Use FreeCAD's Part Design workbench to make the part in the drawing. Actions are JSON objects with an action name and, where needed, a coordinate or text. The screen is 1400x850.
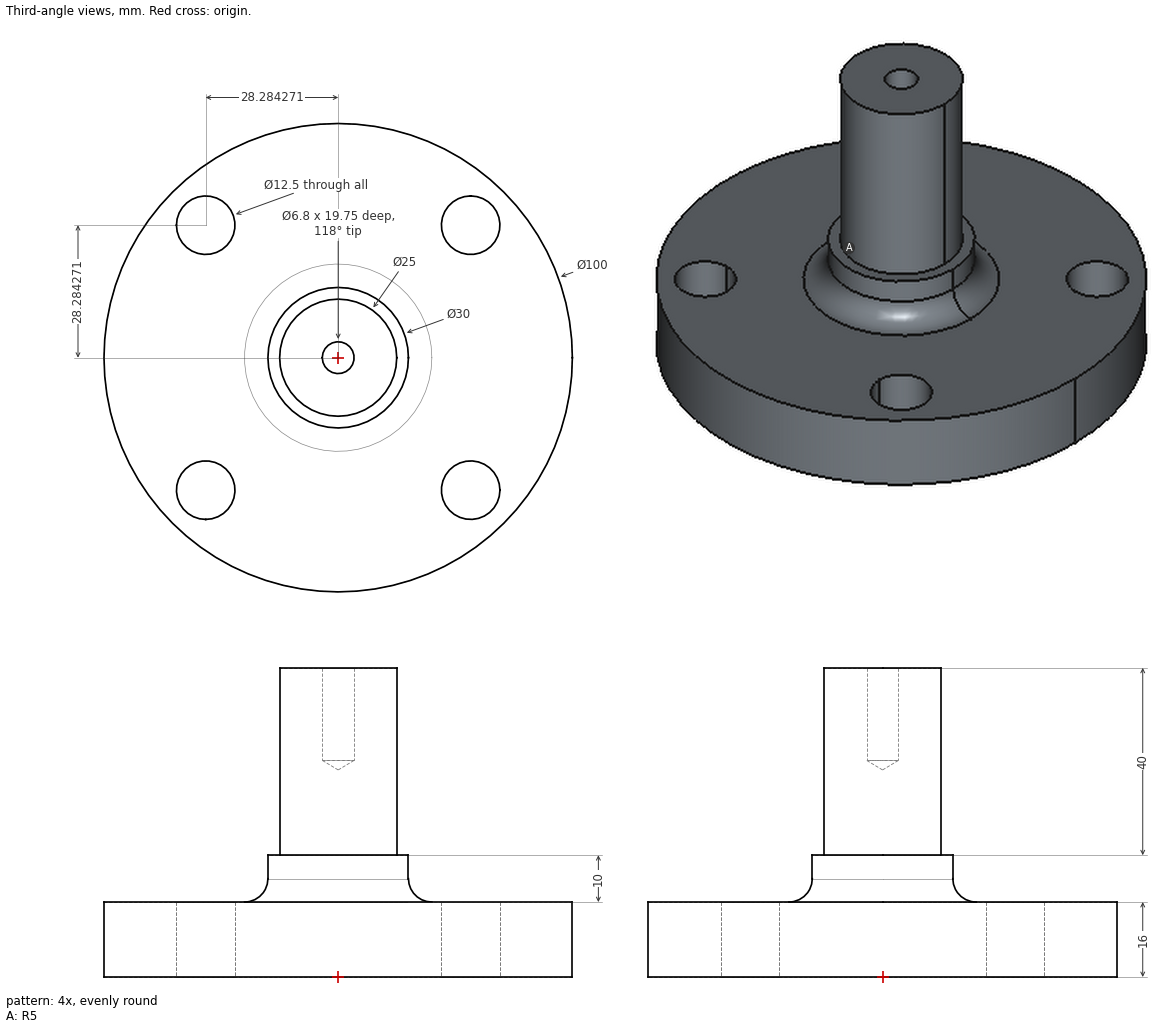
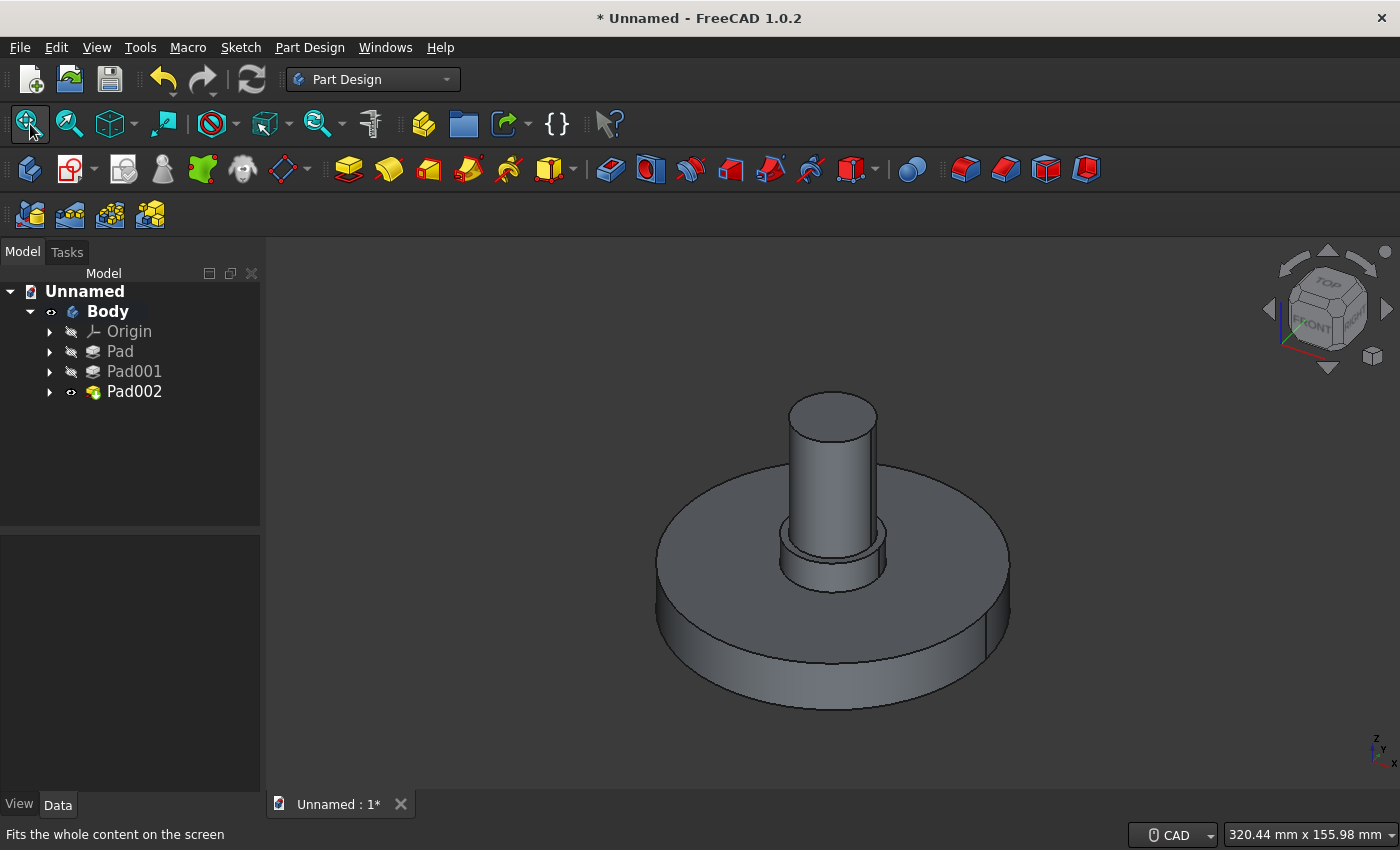
{"action": "left_click", "coordinate": [946, 565]}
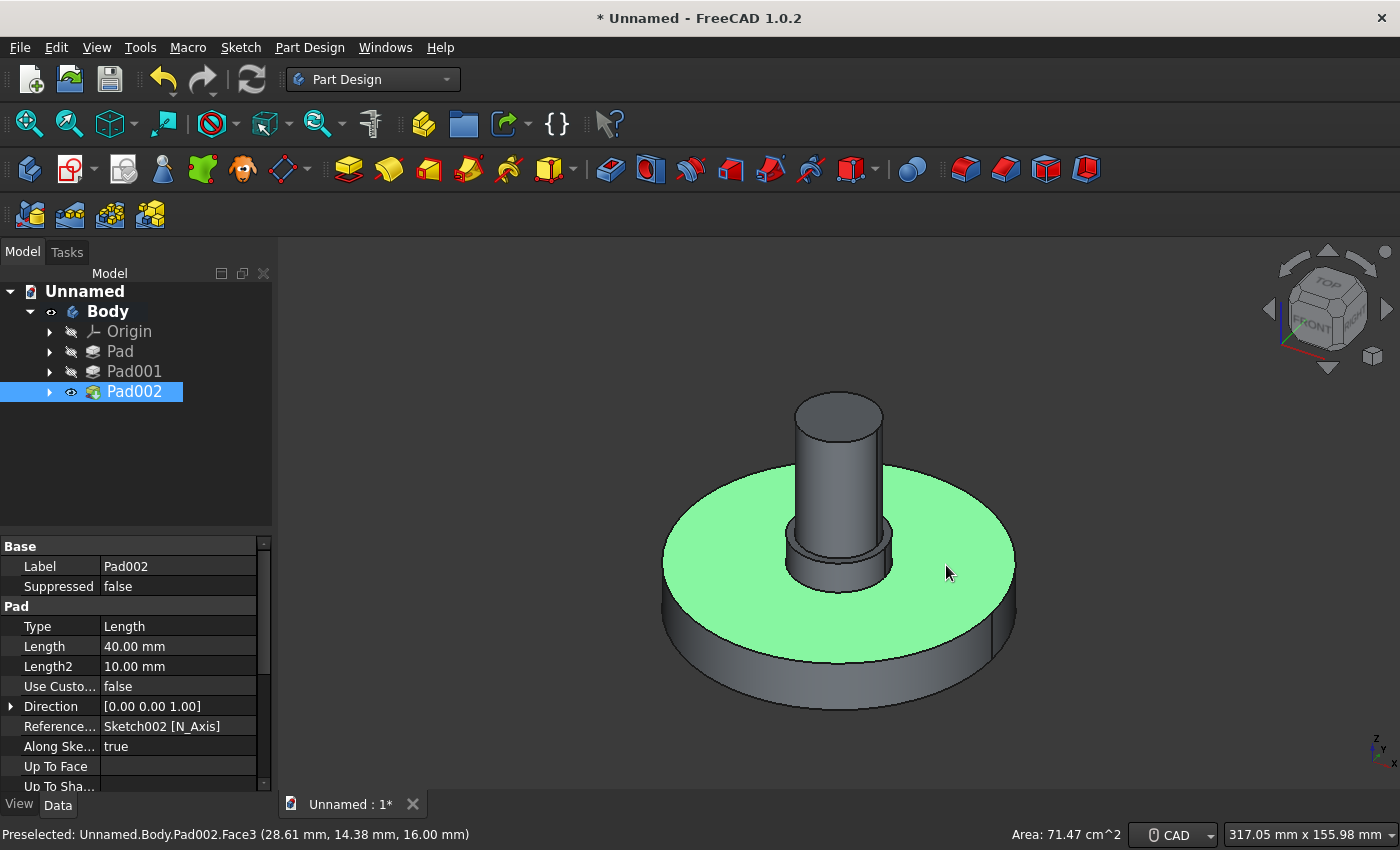
{"action": "left_click", "coordinate": [70, 170]}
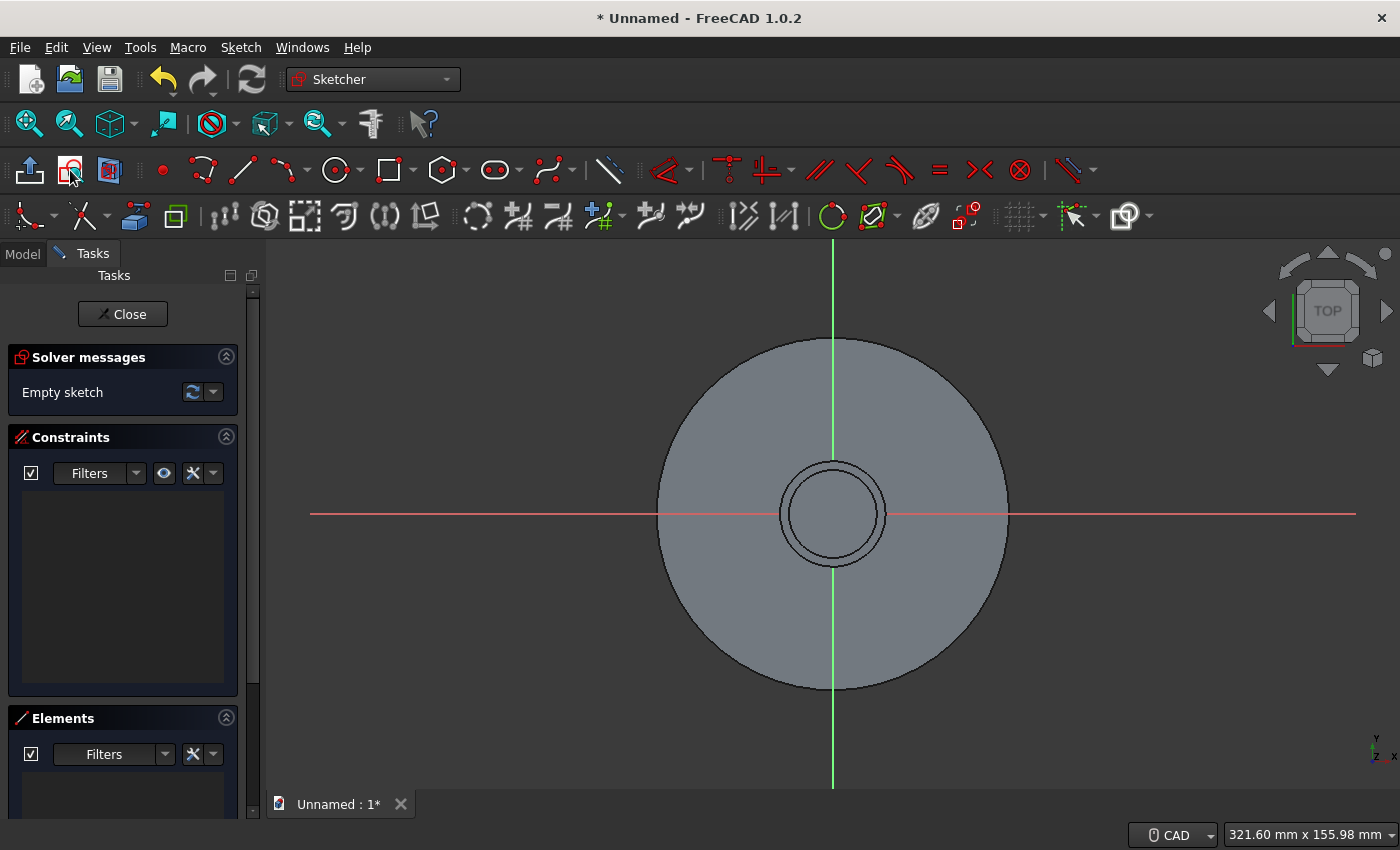
{"action": "scroll", "coordinate": [728, 399], "scroll_direction": "up", "scroll_amount": 10}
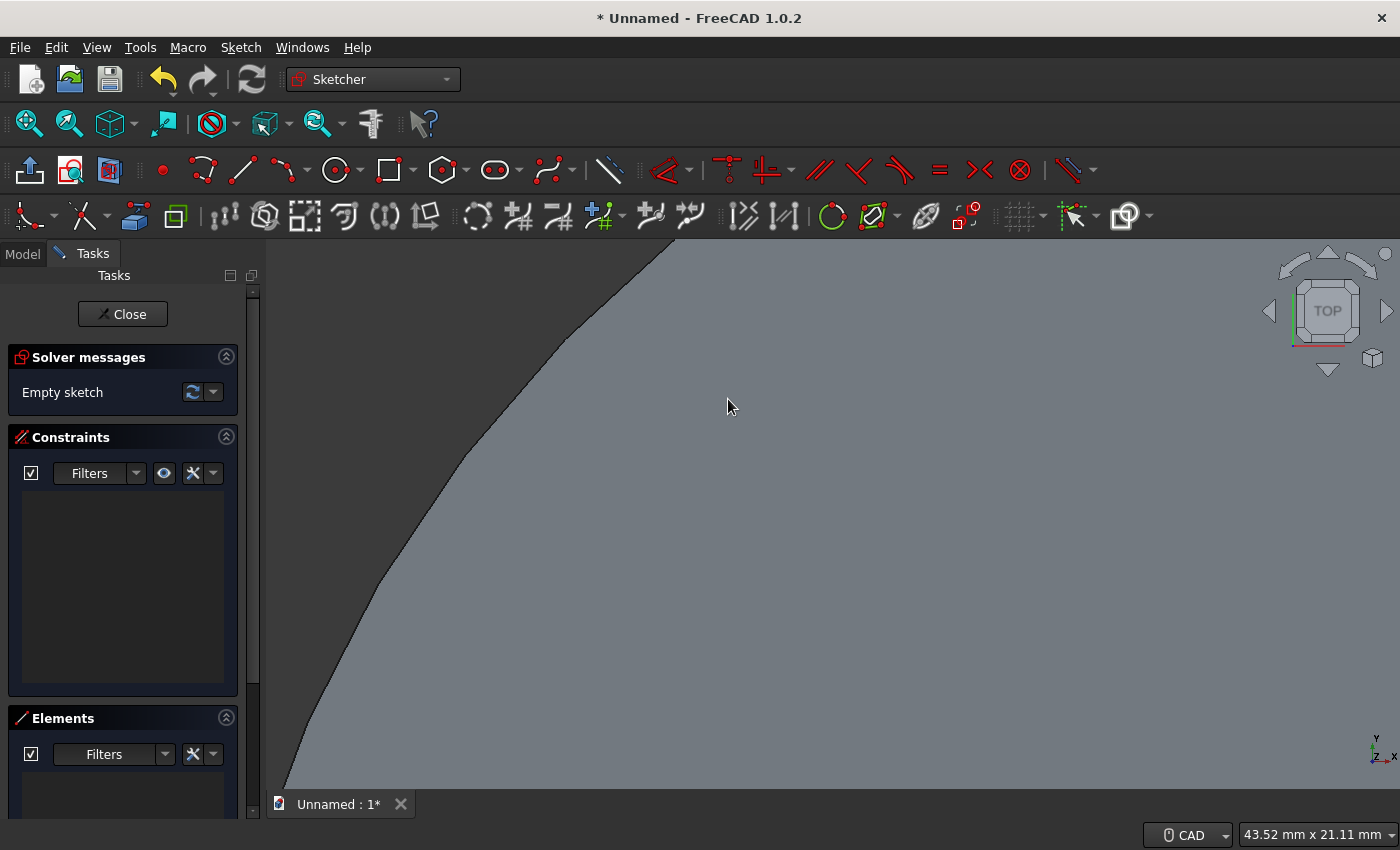
{"action": "key", "text": "g c"}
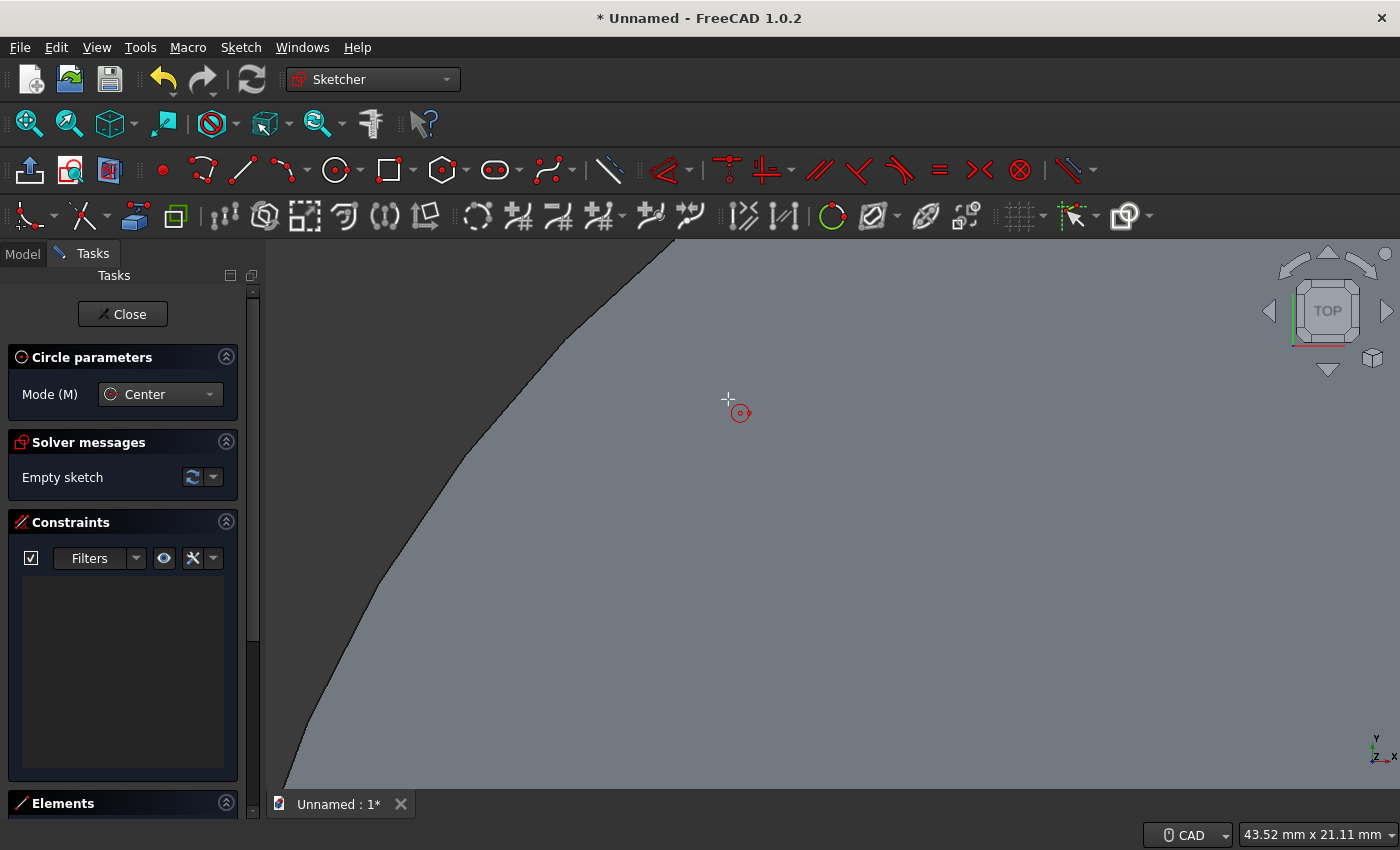
{"action": "left_click", "coordinate": [763, 510]}
{"action": "left_click", "coordinate": [878, 395]}
{"action": "key", "text": "Escape"}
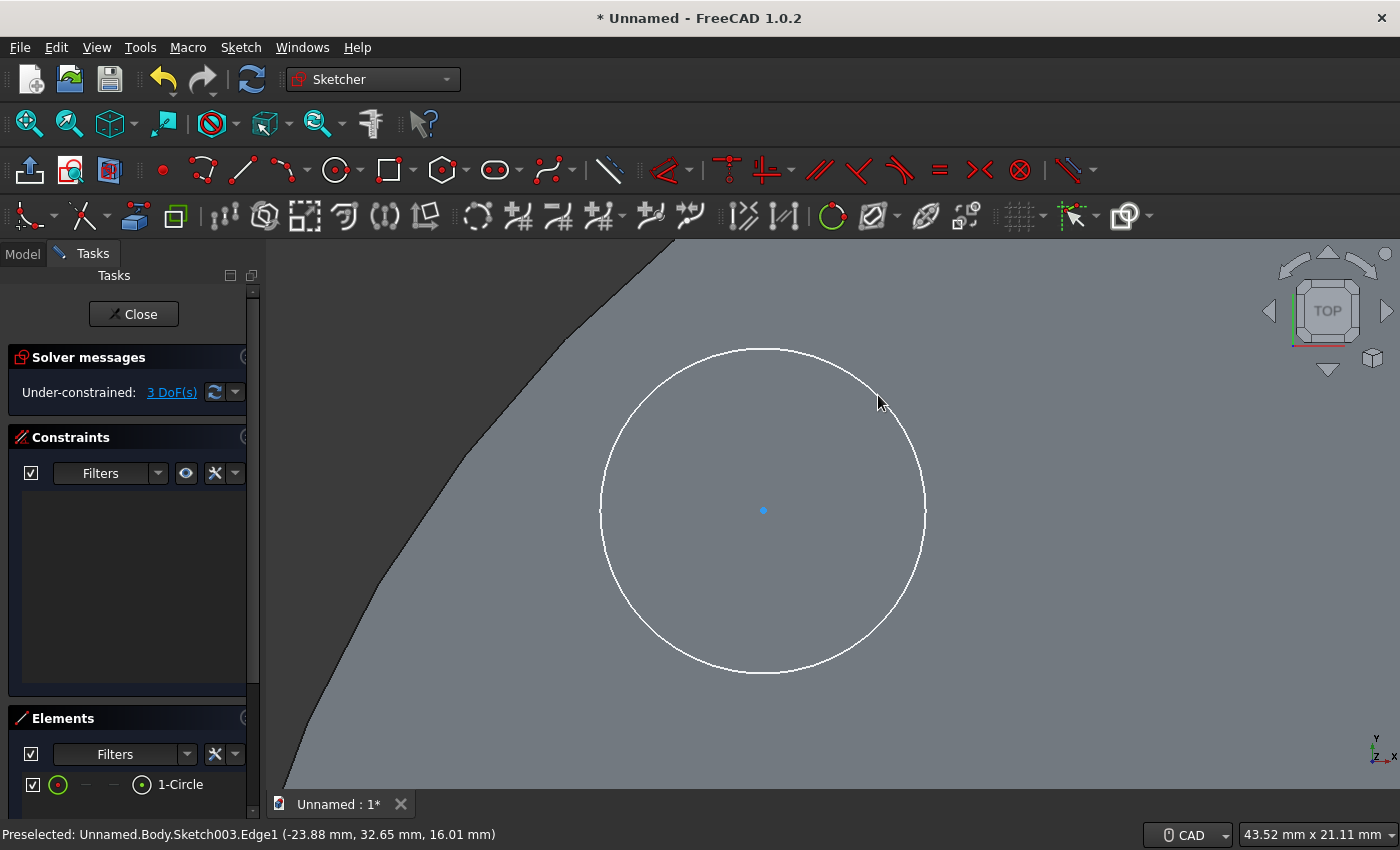
{"action": "key", "text": "d"}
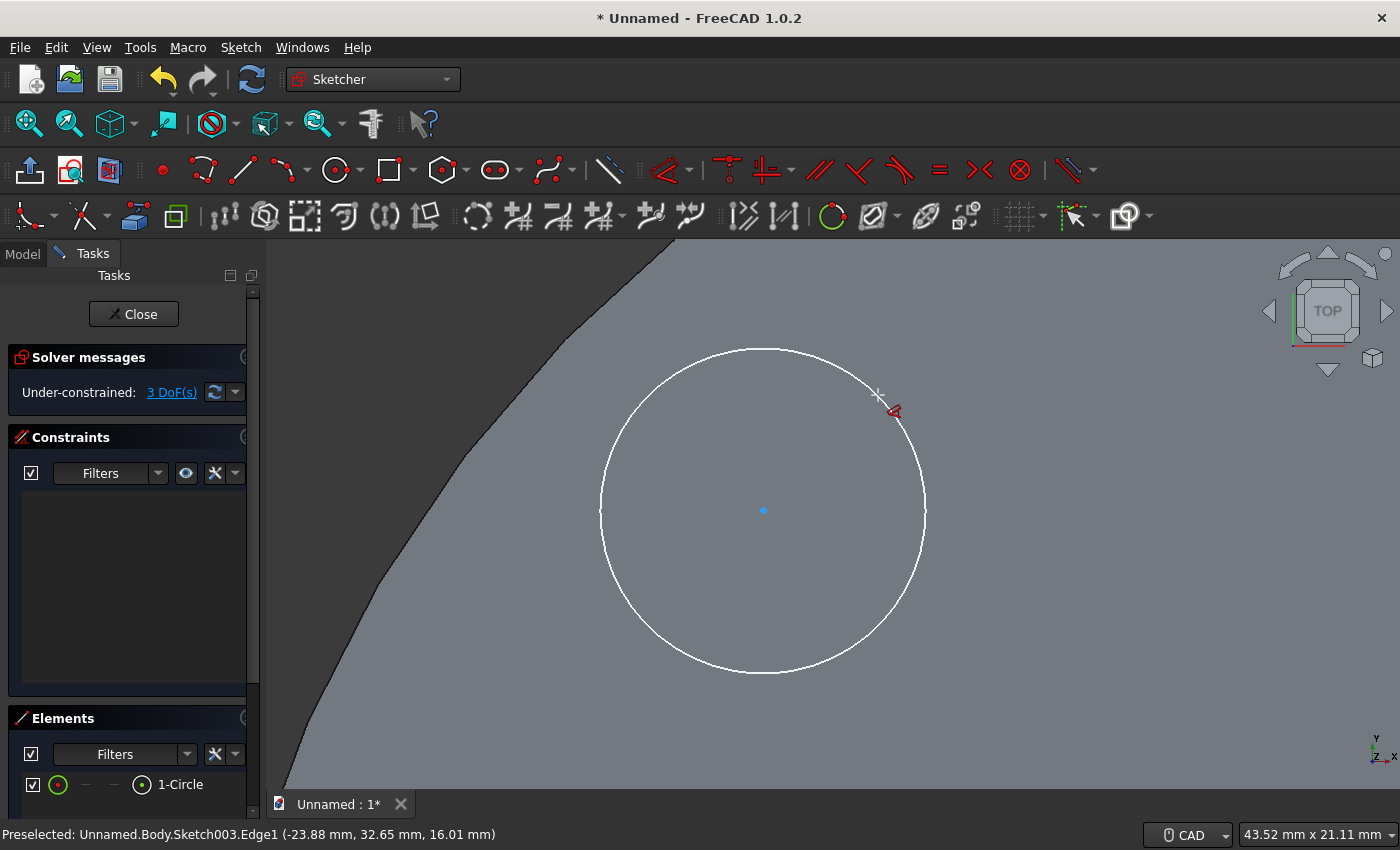
{"action": "left_click", "coordinate": [878, 396]}
{"action": "left_click", "coordinate": [901, 373]}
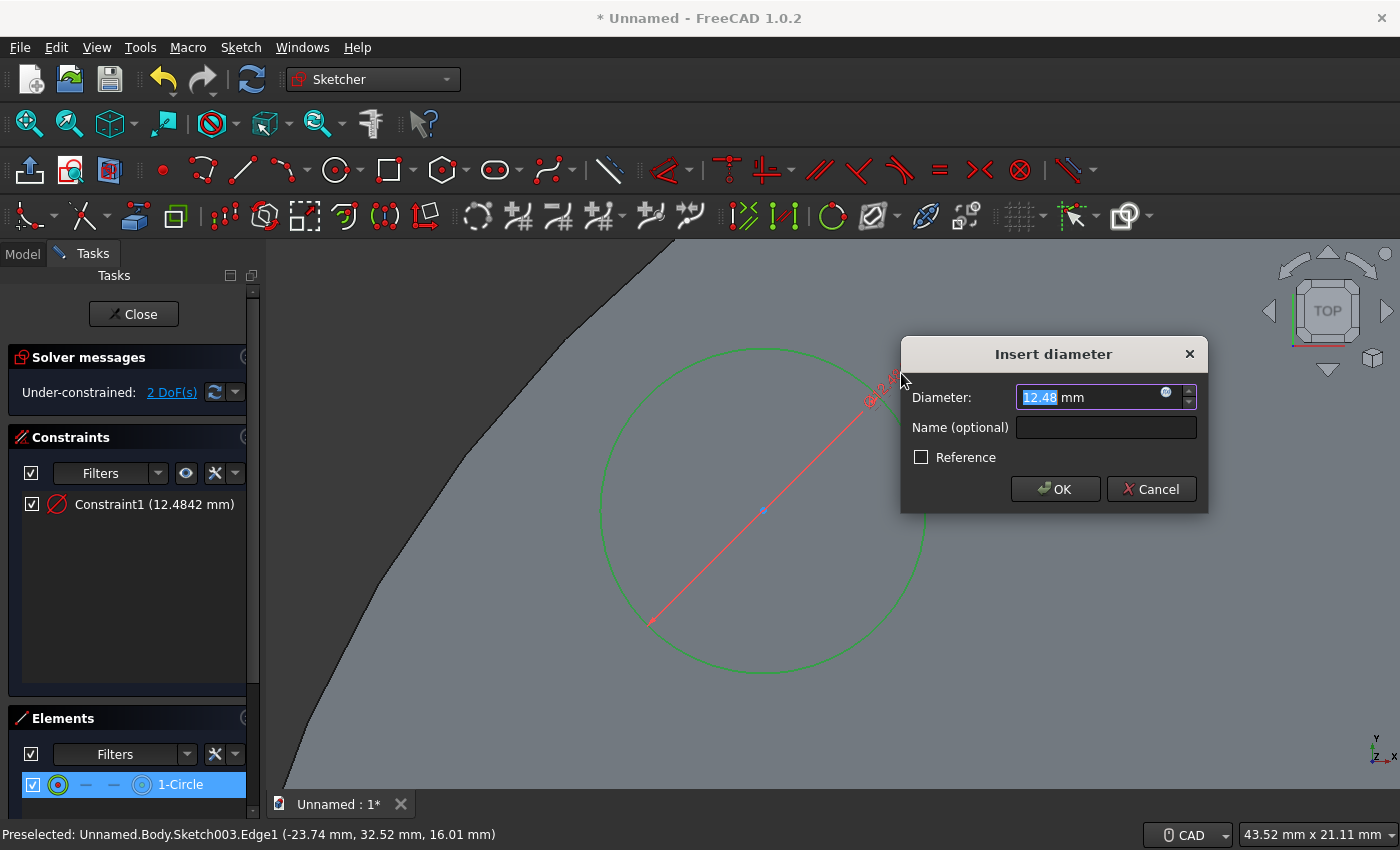
{"action": "type", "text": "12.5"}
{"action": "key", "text": "Return"}